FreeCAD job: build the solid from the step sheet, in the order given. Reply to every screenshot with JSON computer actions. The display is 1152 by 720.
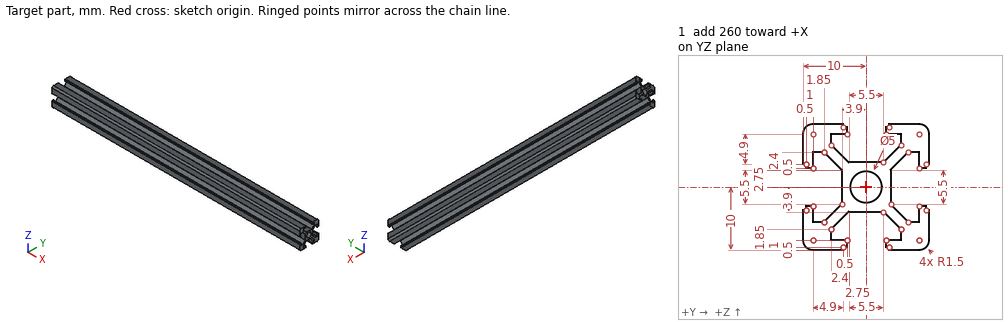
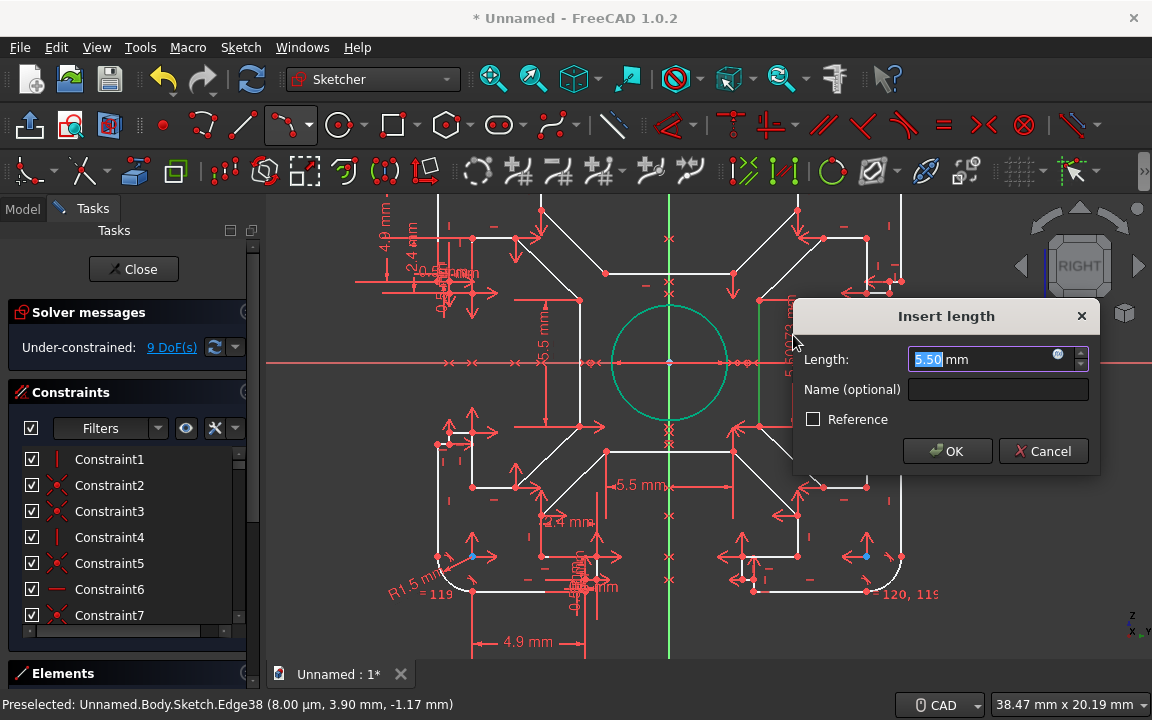
{"action": "type", "text": "5.5"}
{"action": "key", "text": "Return"}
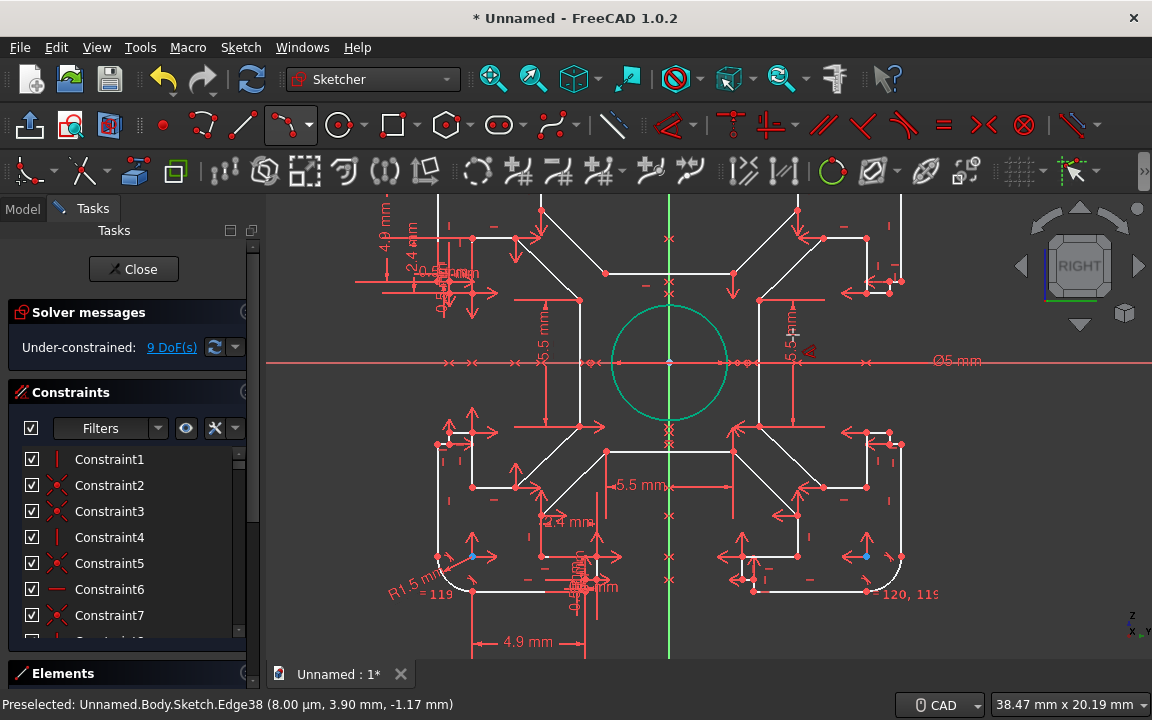
{"action": "left_click", "coordinate": [695, 274]}
{"action": "left_click", "coordinate": [640, 240]}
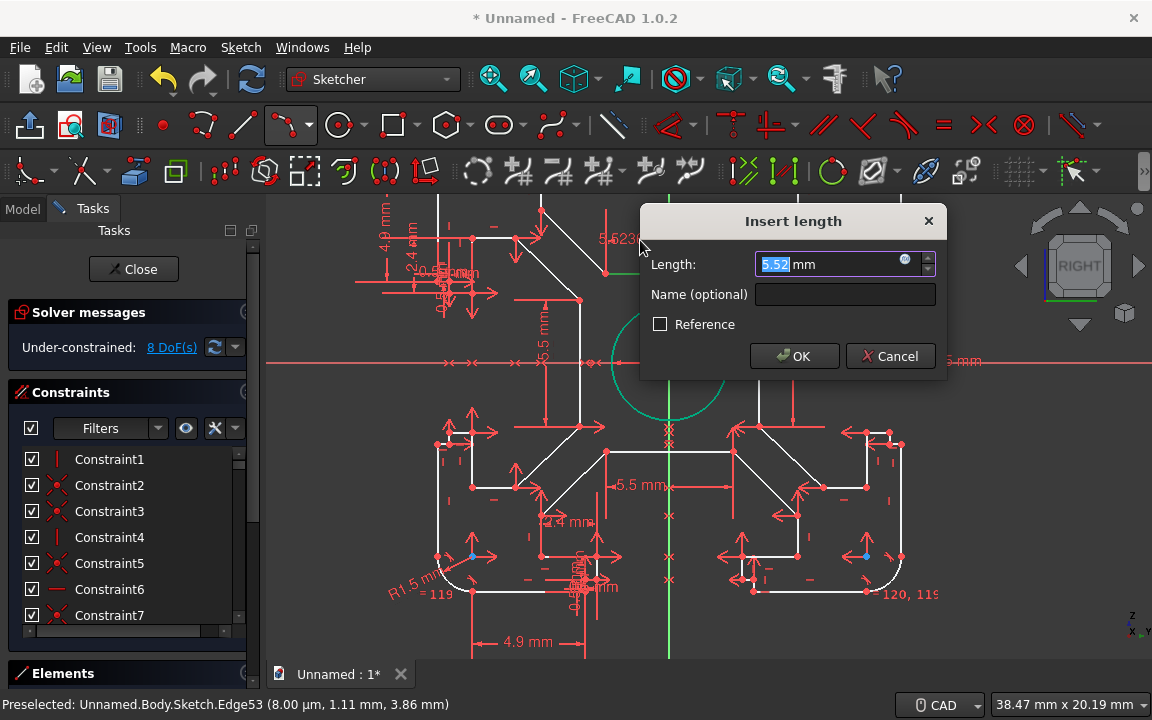
{"action": "type", "text": "5.5"}
{"action": "key", "text": "Return"}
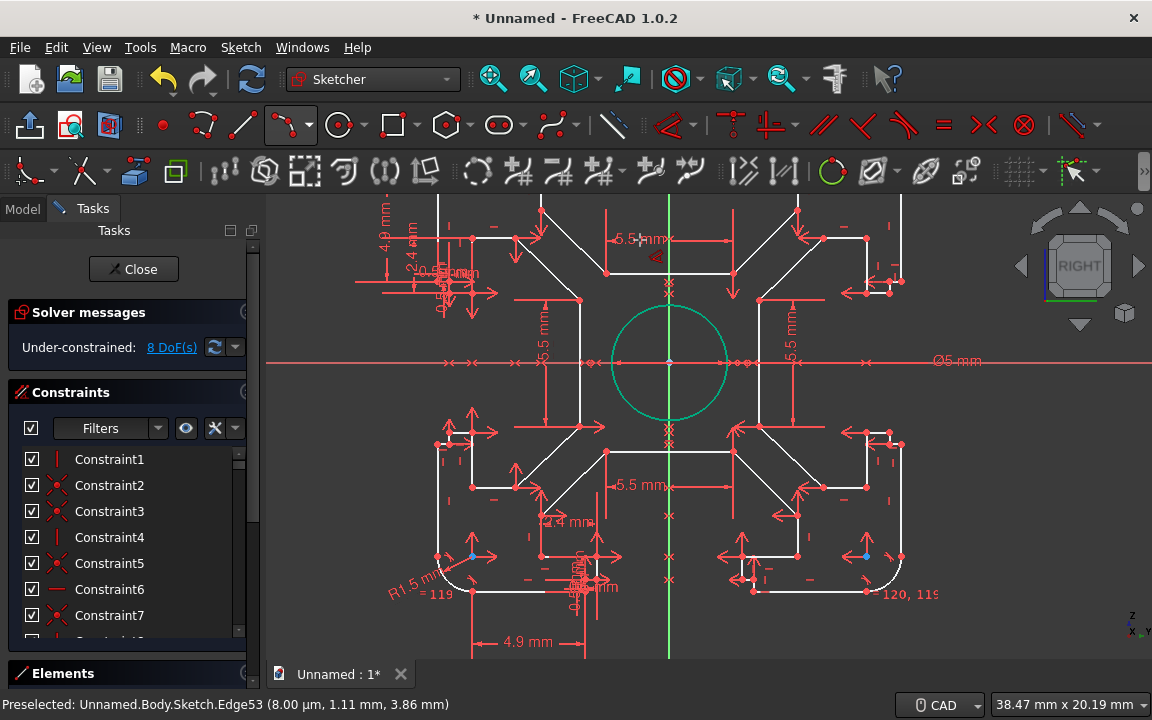
{"action": "left_click", "coordinate": [485, 238]}
{"action": "left_click", "coordinate": [494, 392]}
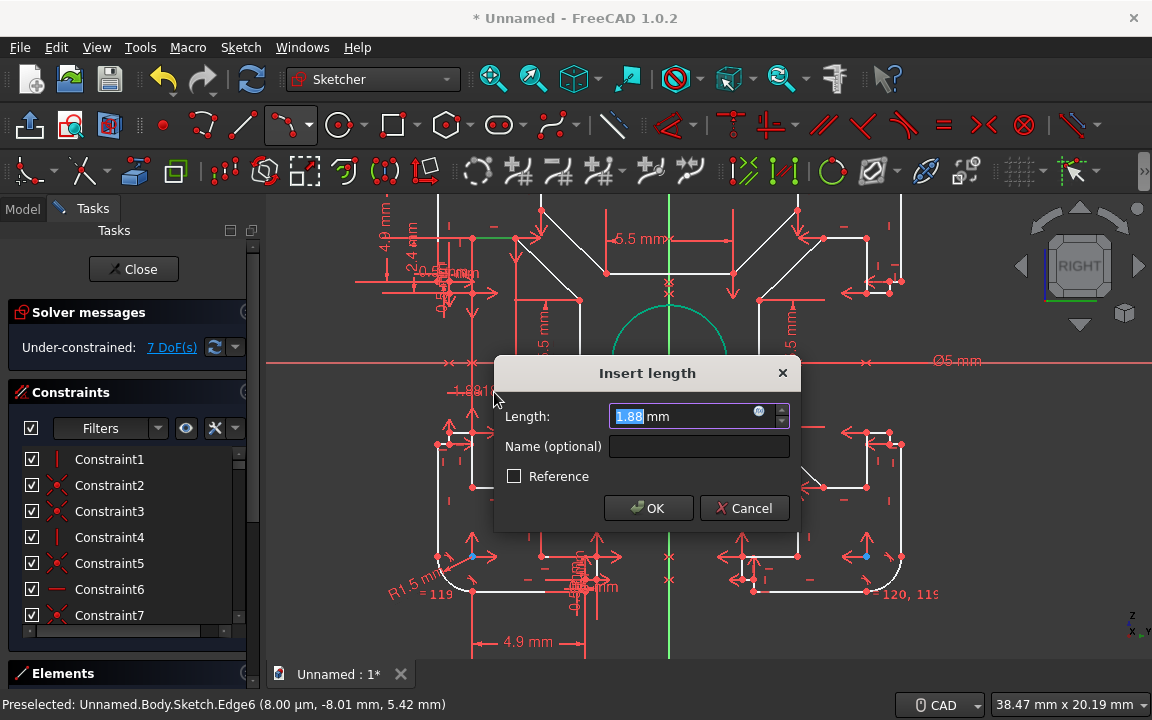
{"action": "type", "text": "1.85"}
{"action": "key", "text": "Return"}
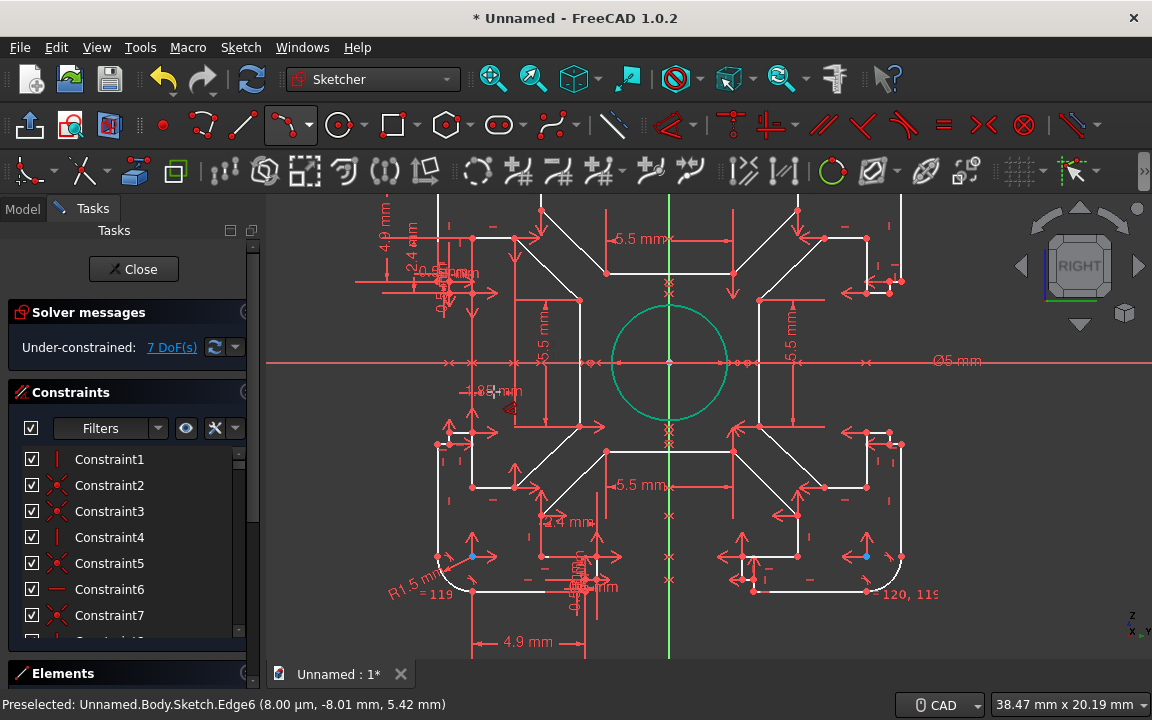
{"action": "left_click", "coordinate": [541, 545]}
{"action": "left_click", "coordinate": [507, 546]}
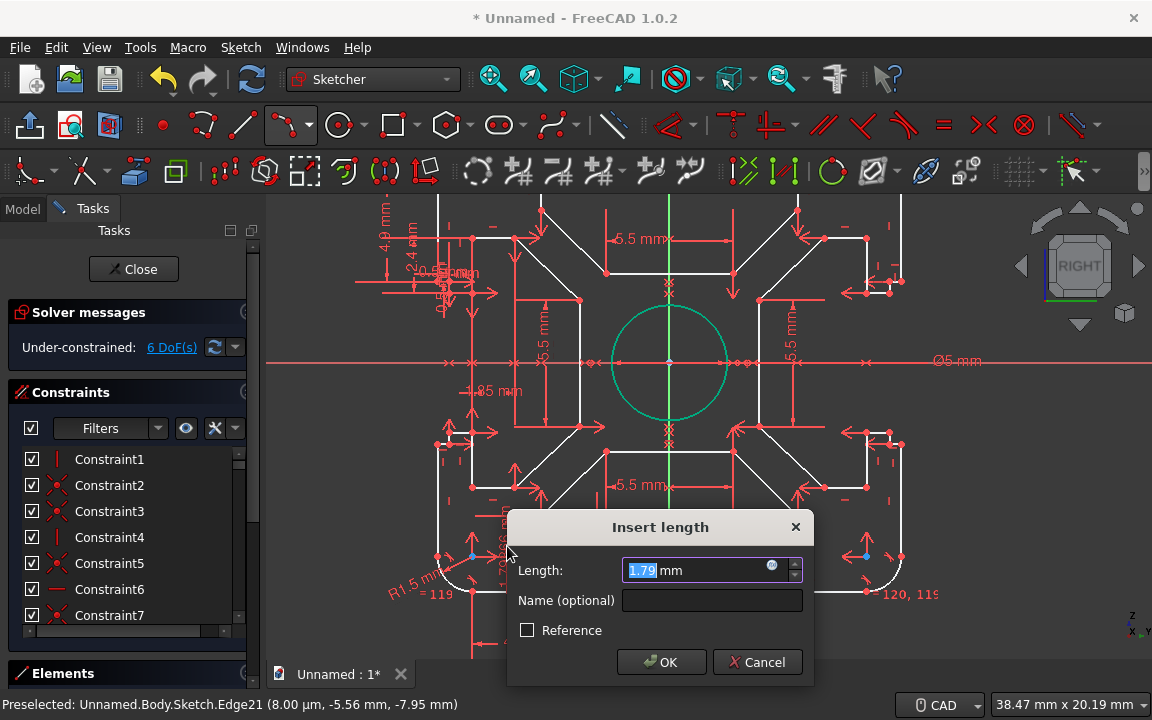
{"action": "type", "text": "1.85"}
{"action": "key", "text": "Return"}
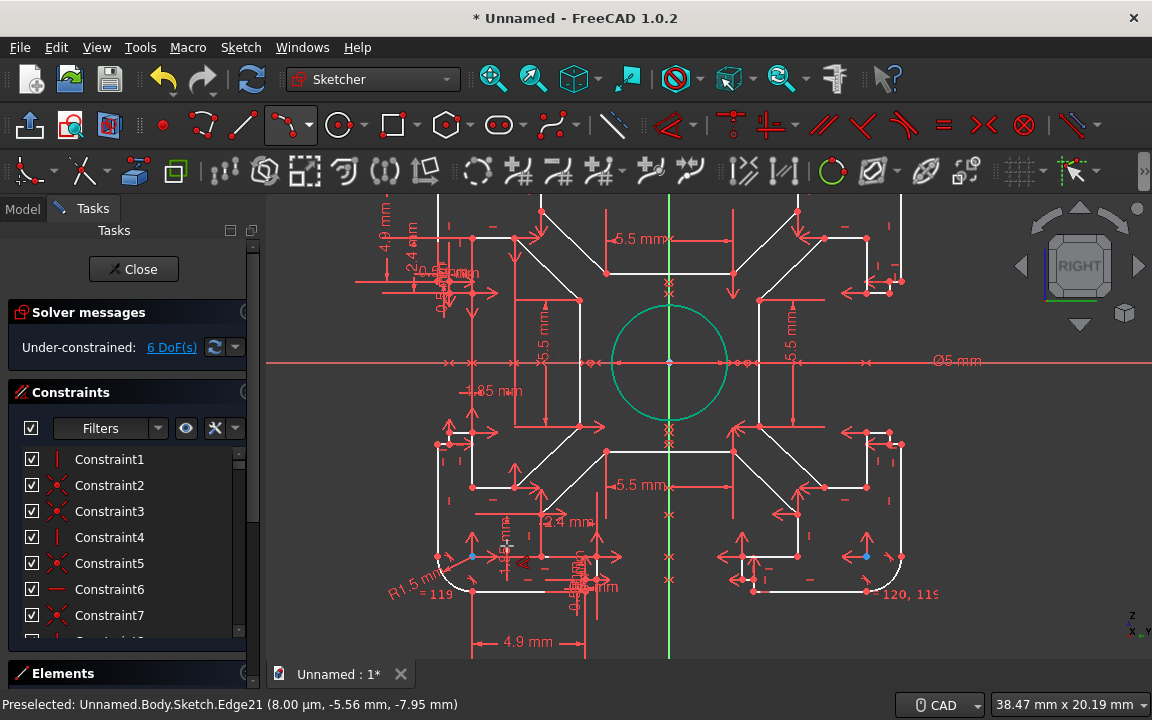
{"action": "left_click", "coordinate": [580, 300]}
{"action": "left_click", "coordinate": [604, 397]}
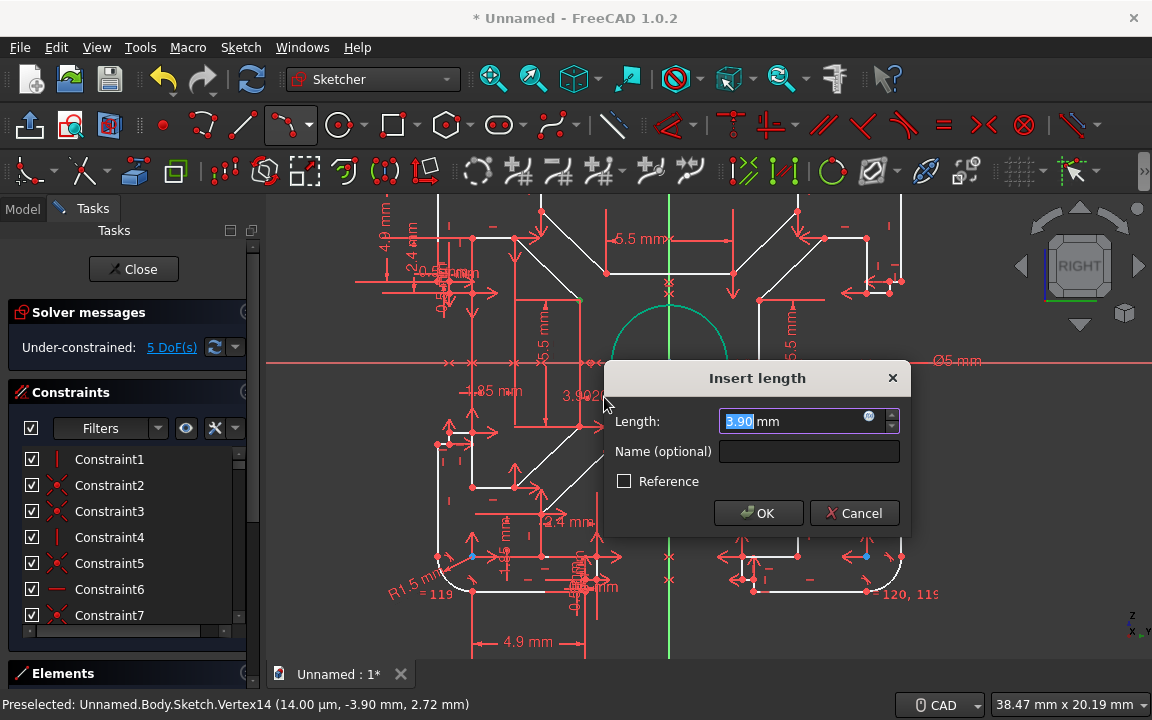
{"action": "type", "text": "3.9"}
{"action": "key", "text": "Return"}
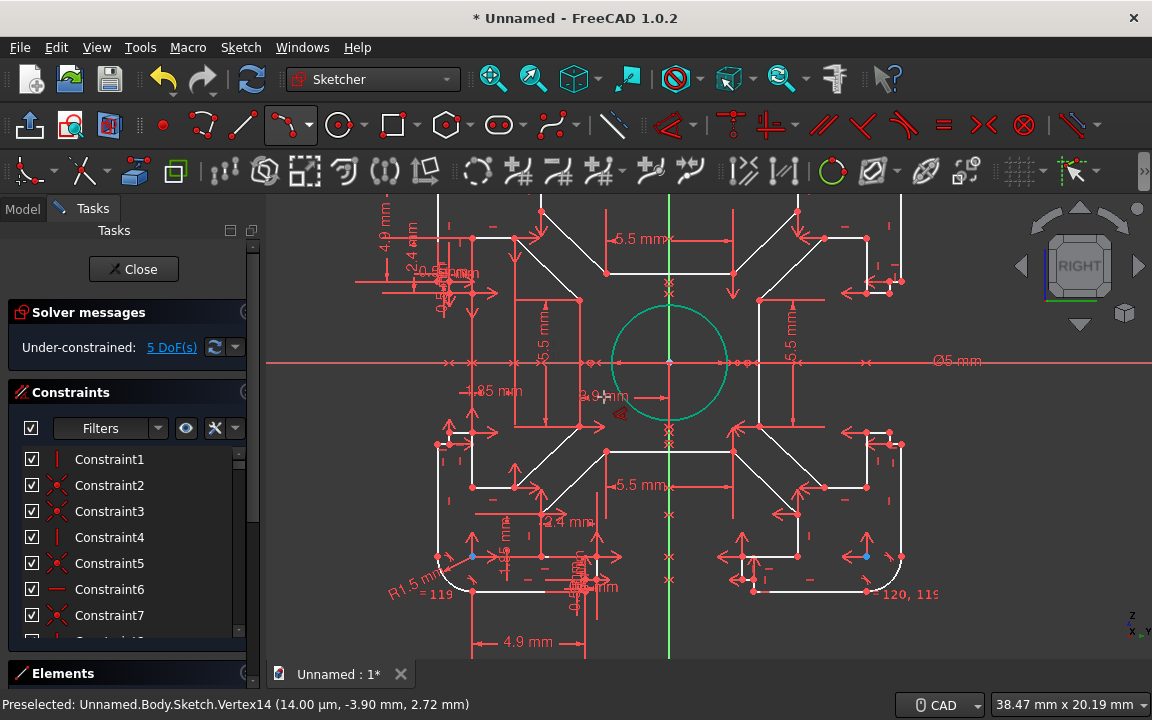
{"action": "left_click", "coordinate": [606, 452]}
{"action": "left_click", "coordinate": [703, 387]}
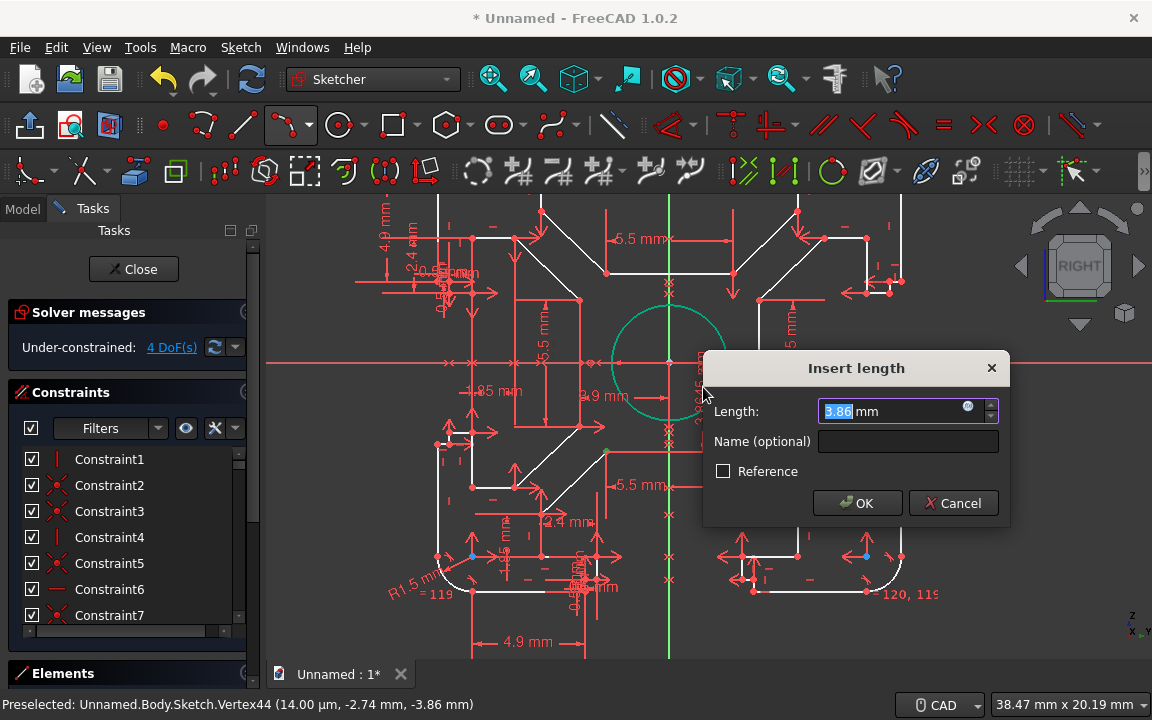
{"action": "type", "text": "3.9"}
{"action": "key", "text": "Return"}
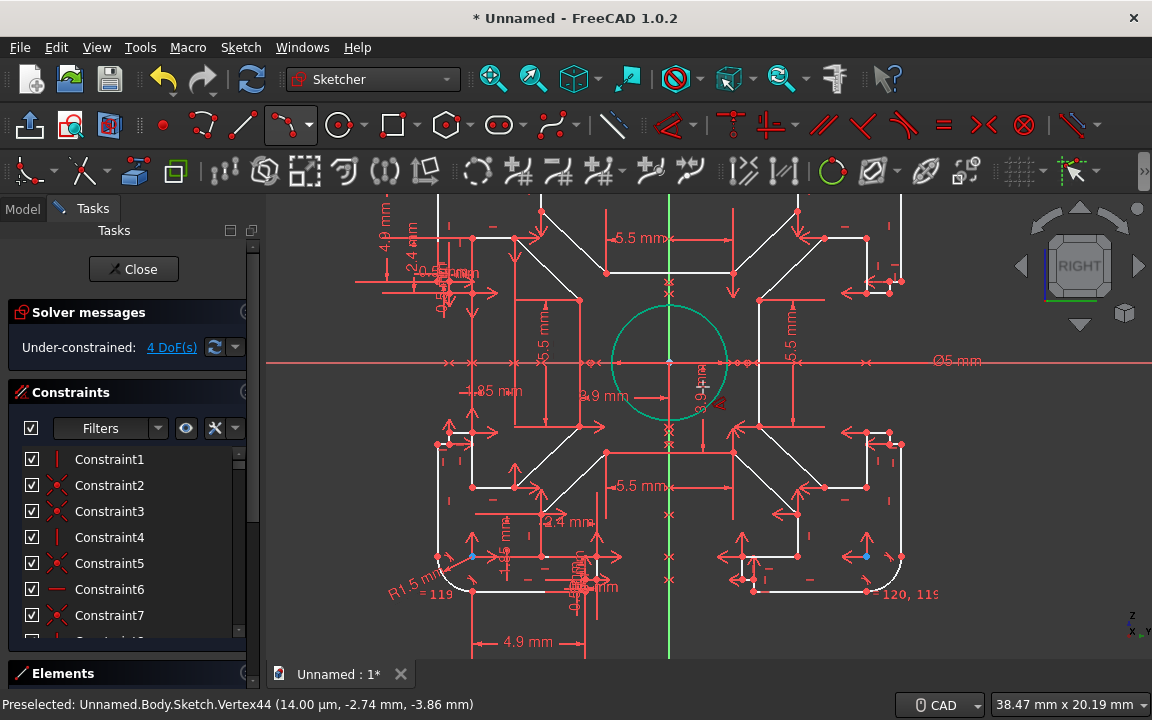
{"action": "left_click", "coordinate": [580, 300]}
{"action": "left_click", "coordinate": [546, 310]}